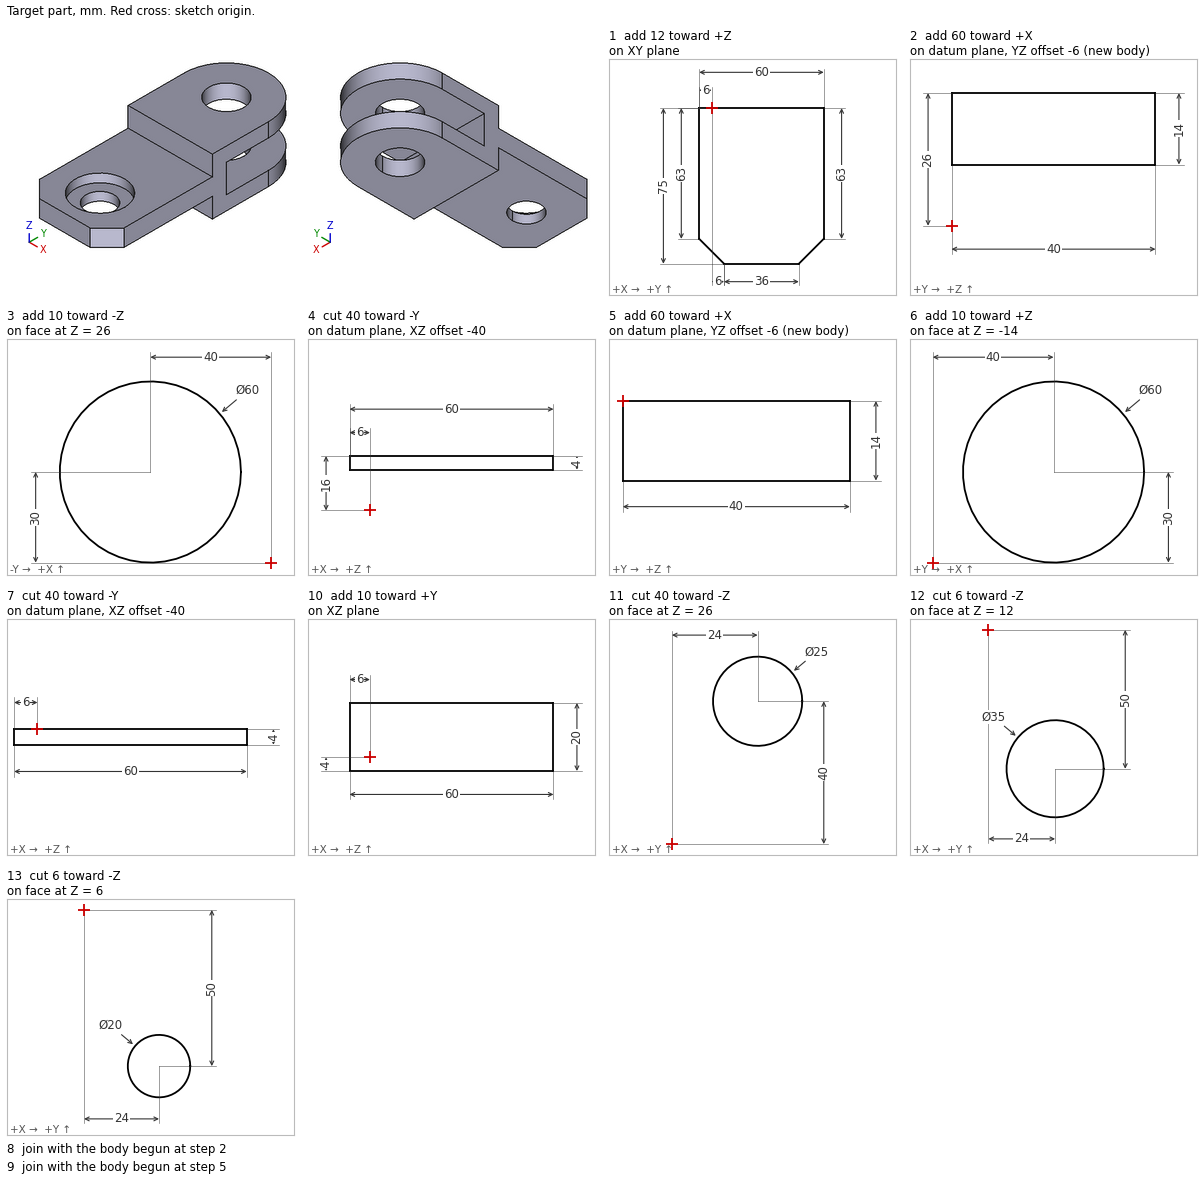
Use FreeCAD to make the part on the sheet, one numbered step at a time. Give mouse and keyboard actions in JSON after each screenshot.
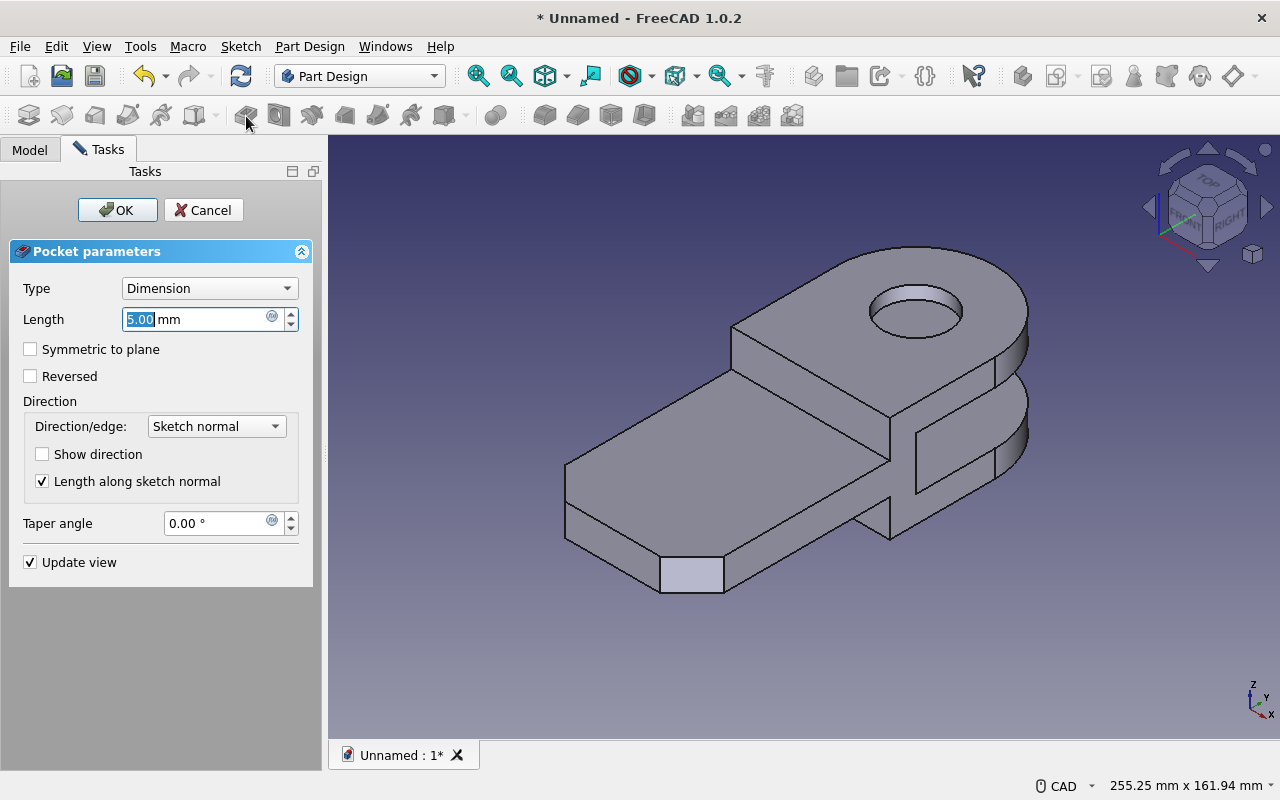
{"action": "type", "text": "40"}
{"action": "key", "text": "Tab"}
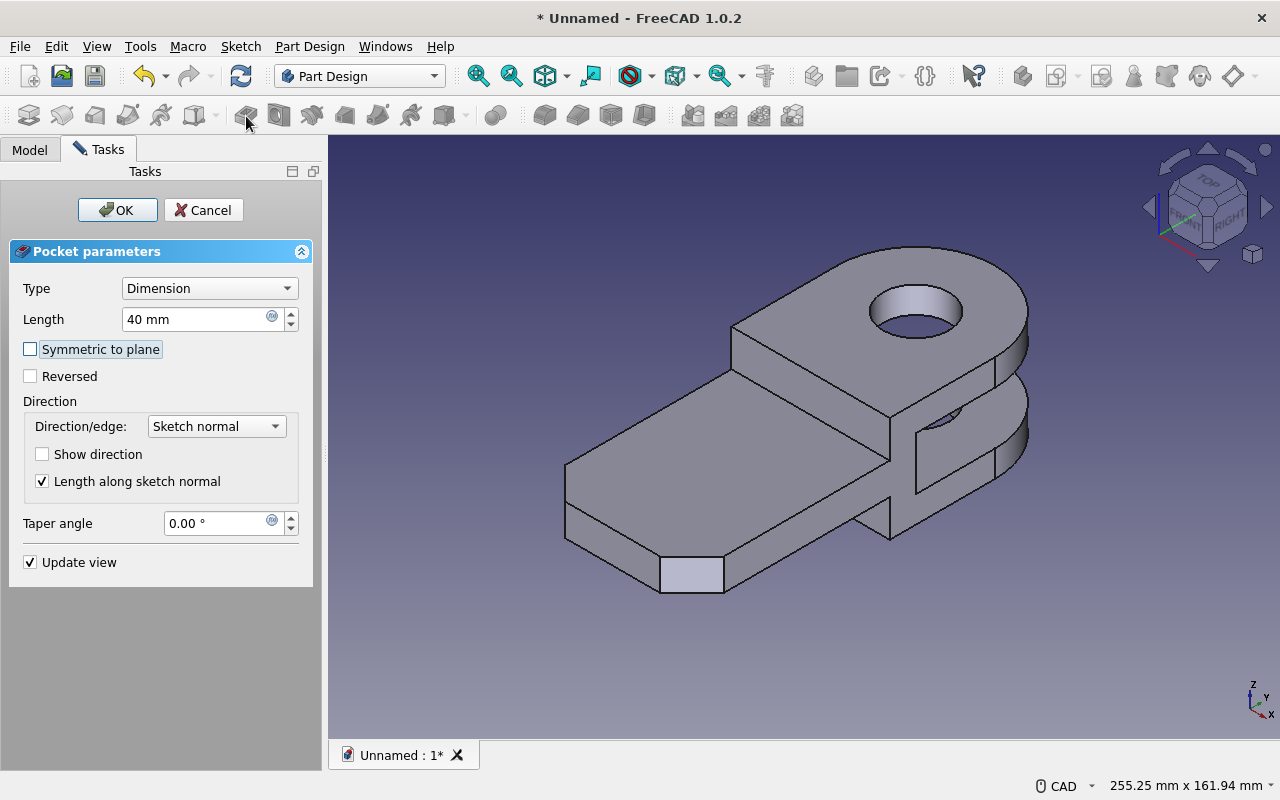
{"action": "left_click", "coordinate": [118, 210]}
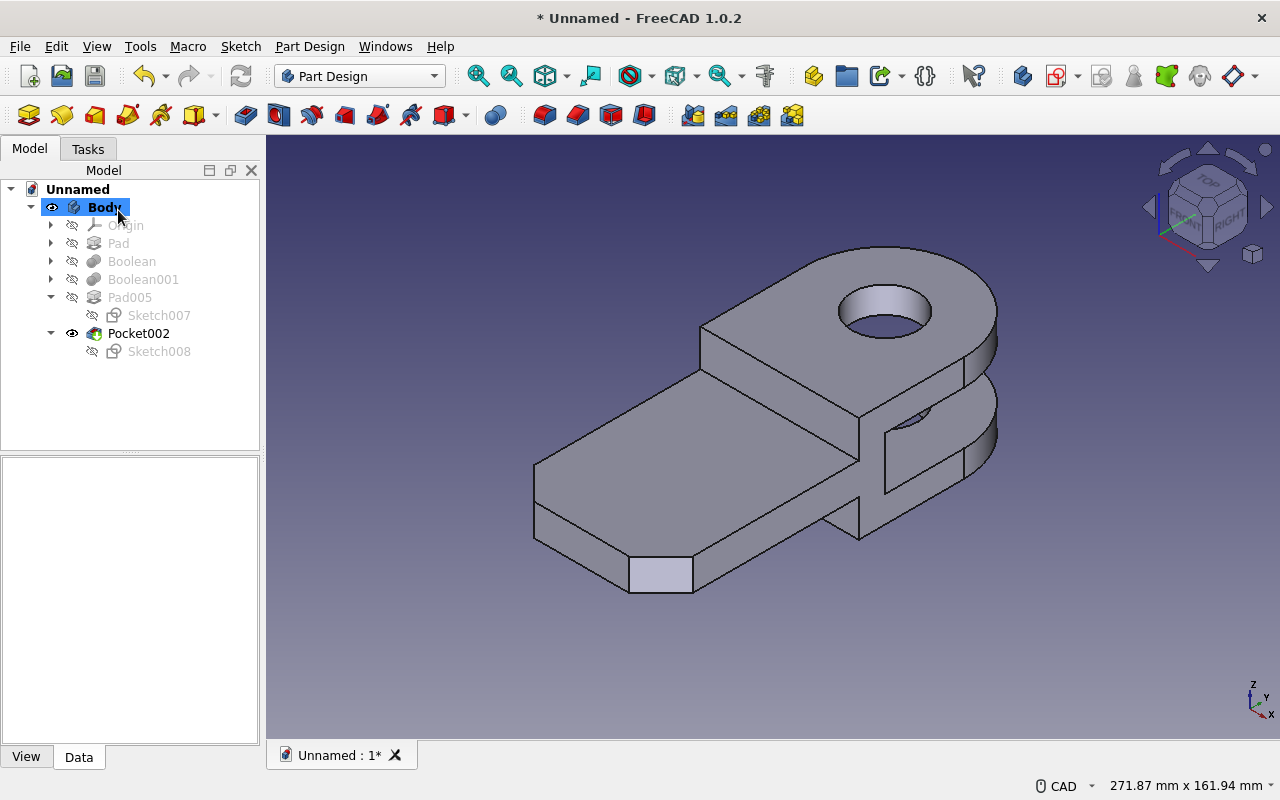
{"action": "left_click", "coordinate": [681, 471]}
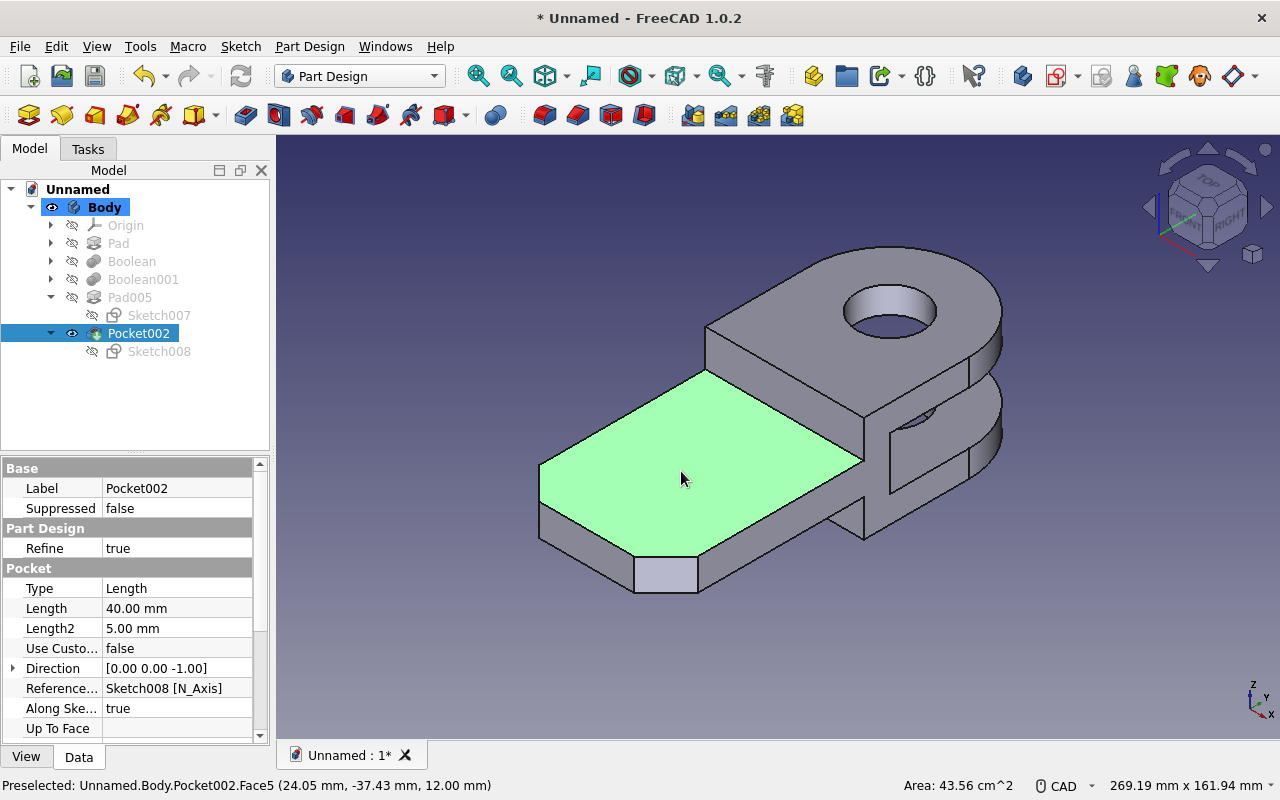
{"action": "left_click", "coordinate": [1056, 76]}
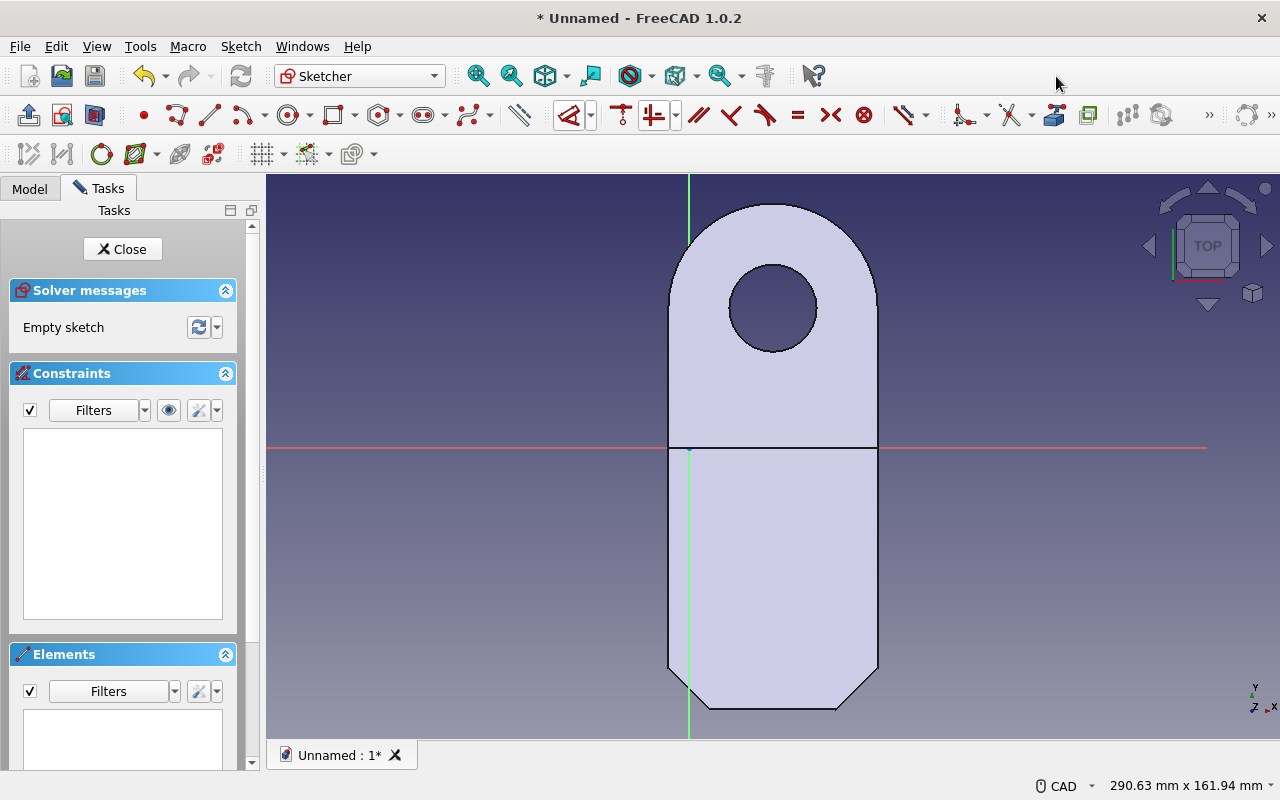
{"action": "scroll", "coordinate": [878, 711], "scroll_direction": "up", "scroll_amount": 2}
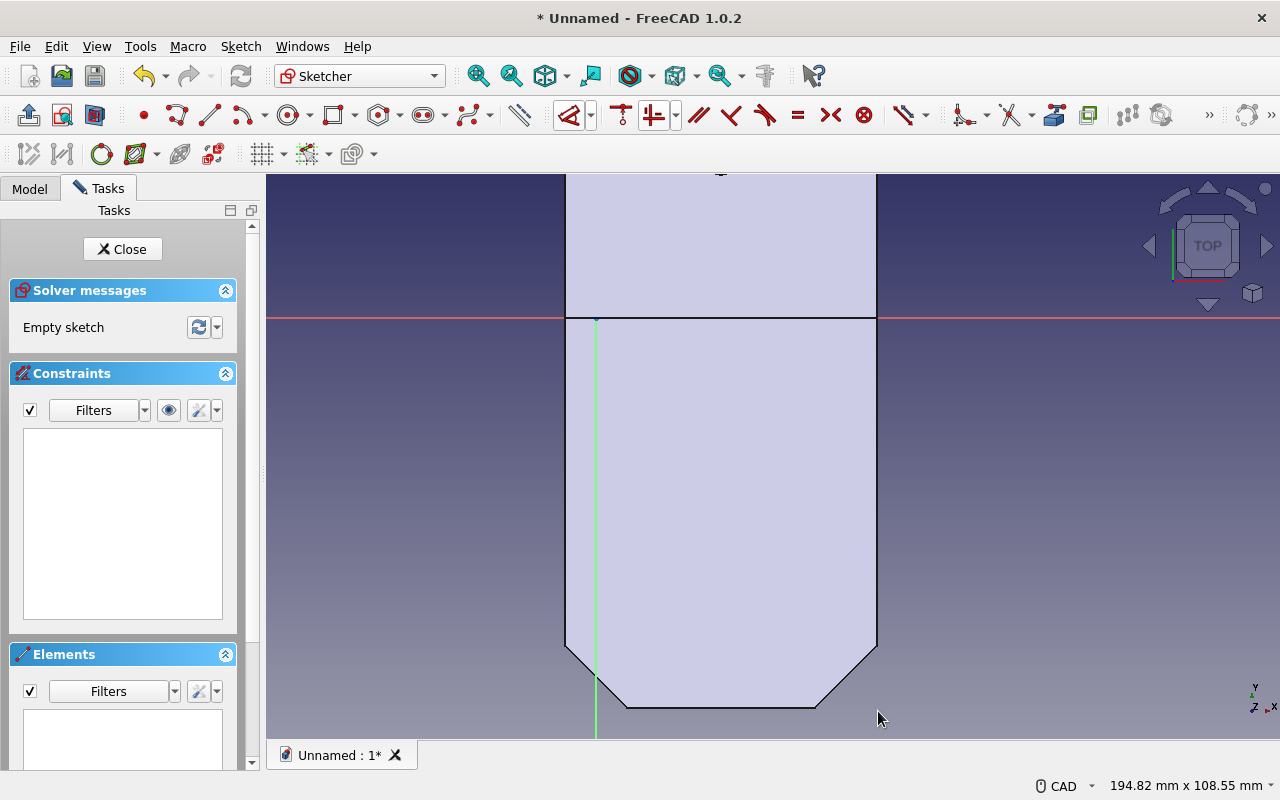
{"action": "left_click", "coordinate": [288, 116]}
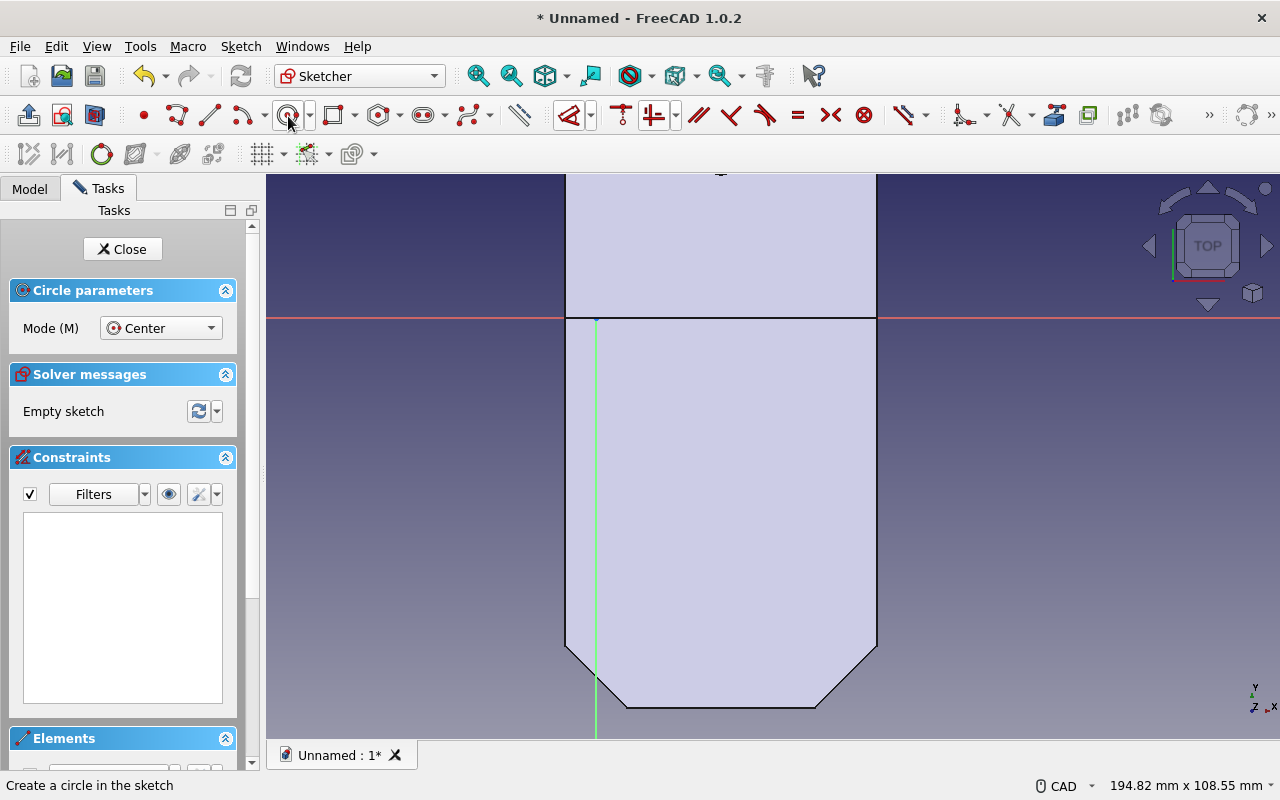
{"action": "left_click", "coordinate": [721, 578]}
{"action": "mouse_move", "coordinate": [785, 514]}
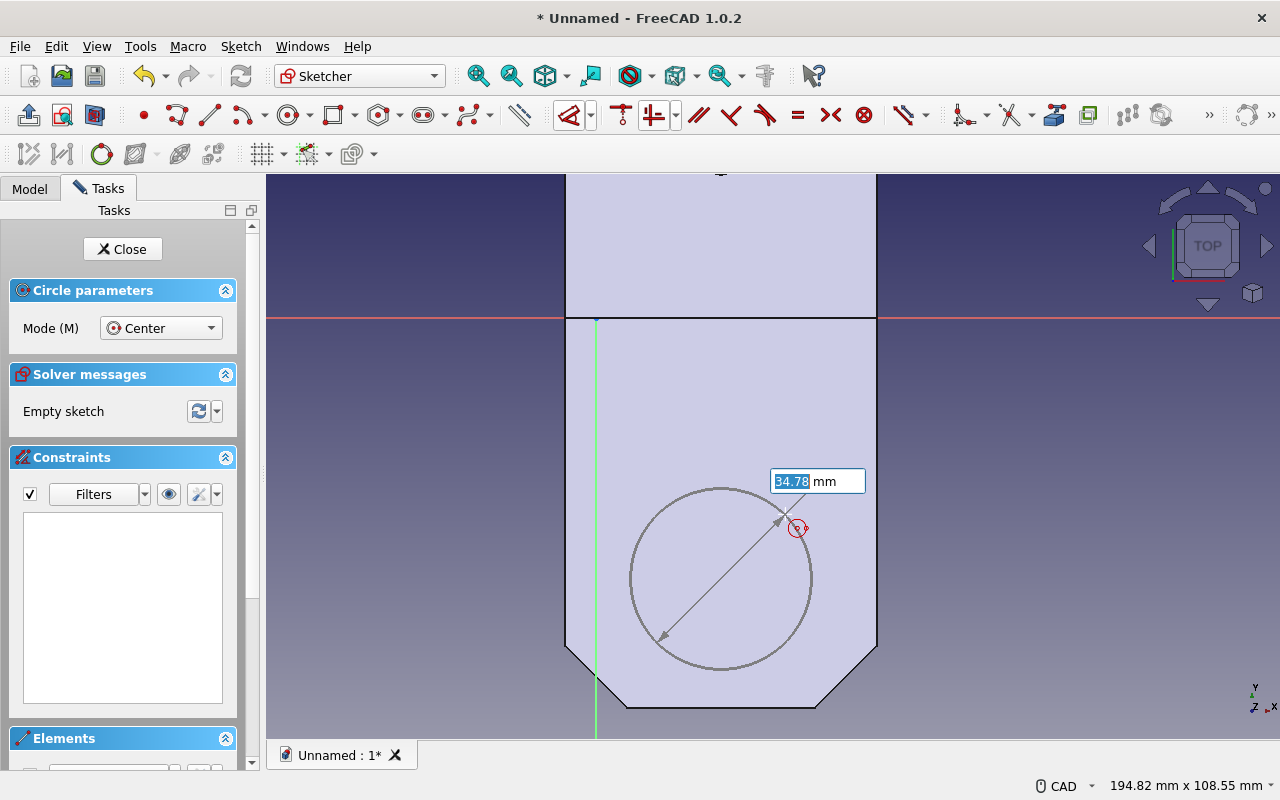
{"action": "type", "text": "35"}
{"action": "key", "text": "Return"}
{"action": "key", "text": "Escape"}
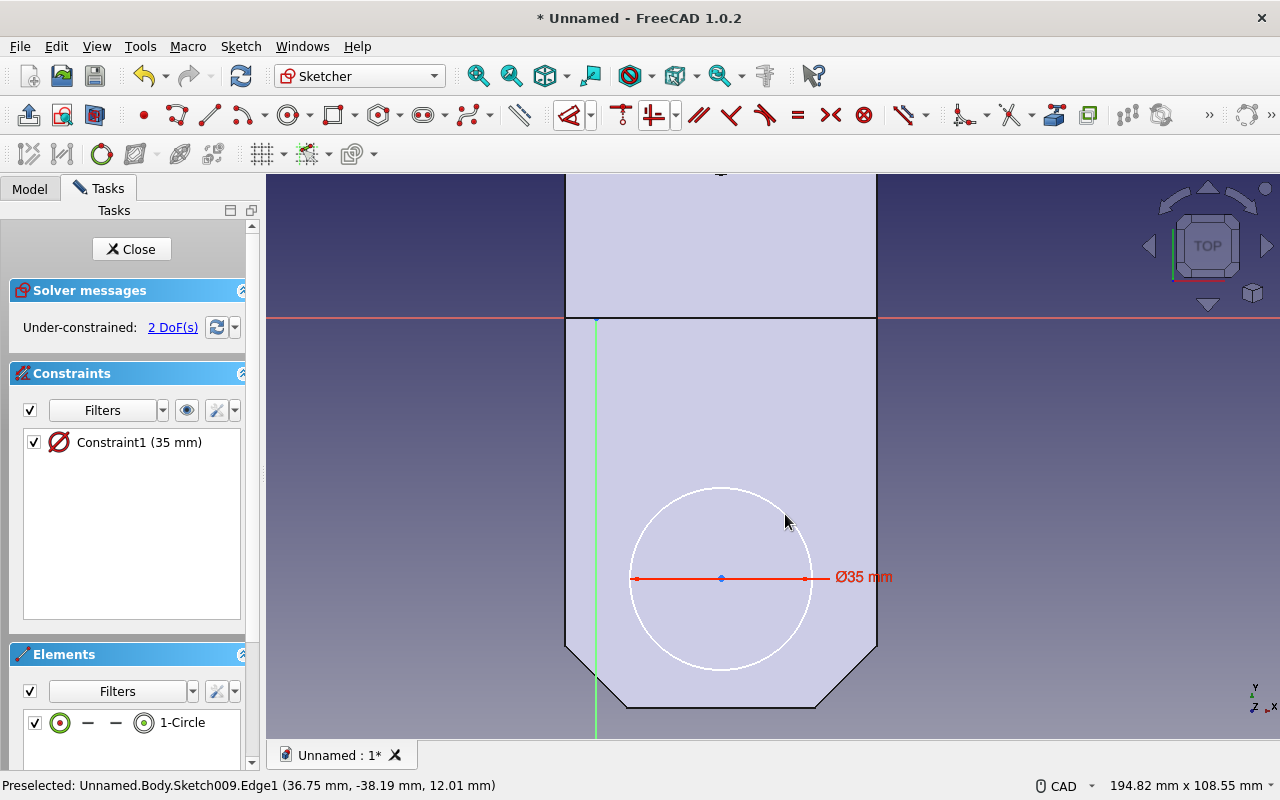
{"action": "left_click", "coordinate": [721, 579]}